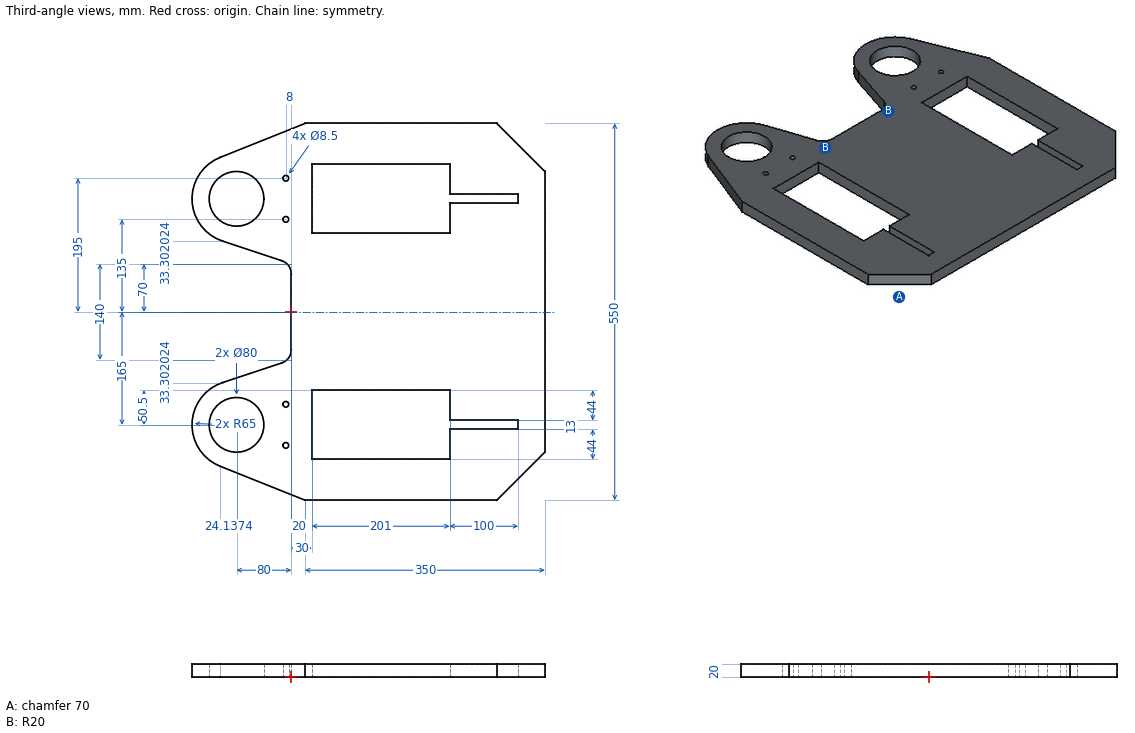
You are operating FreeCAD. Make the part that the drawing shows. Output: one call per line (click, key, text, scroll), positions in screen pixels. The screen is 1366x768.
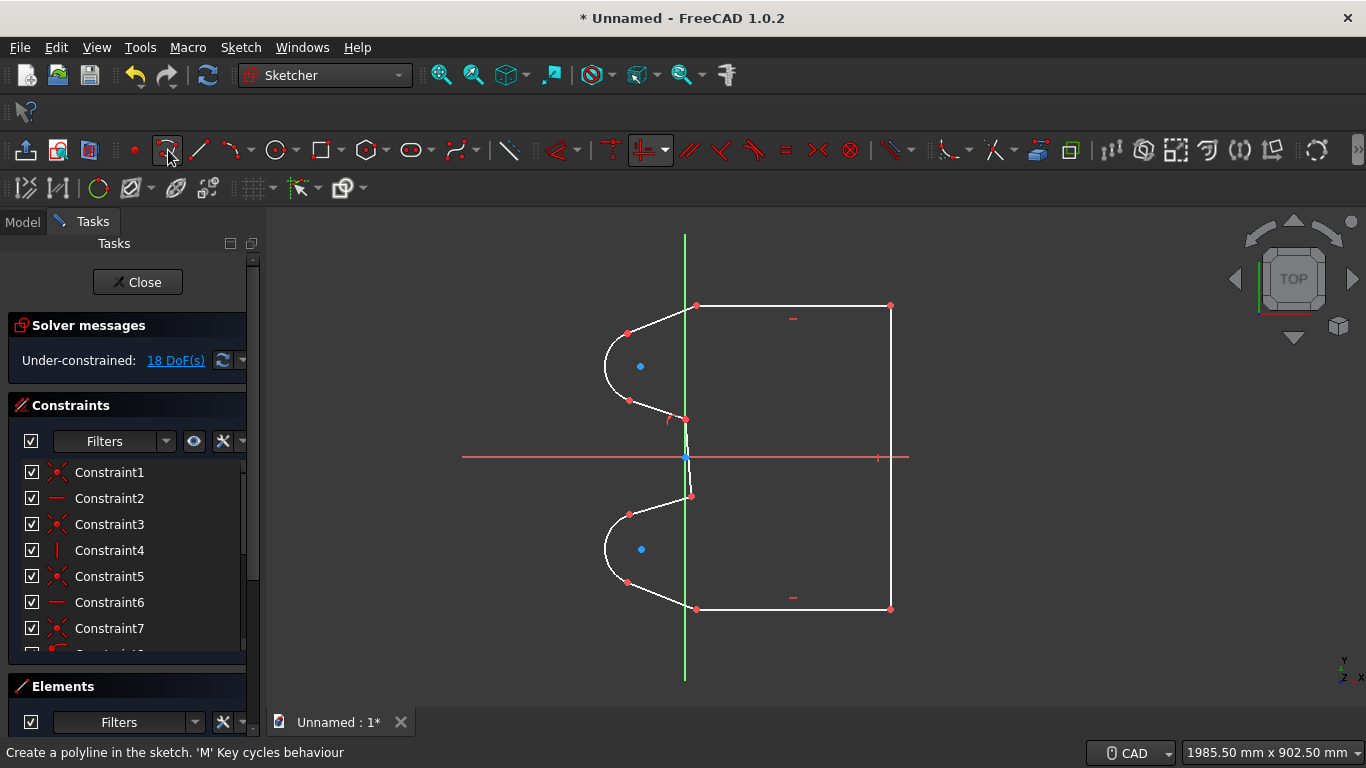
click(702, 521)
click(813, 521)
click(813, 545)
click(869, 545)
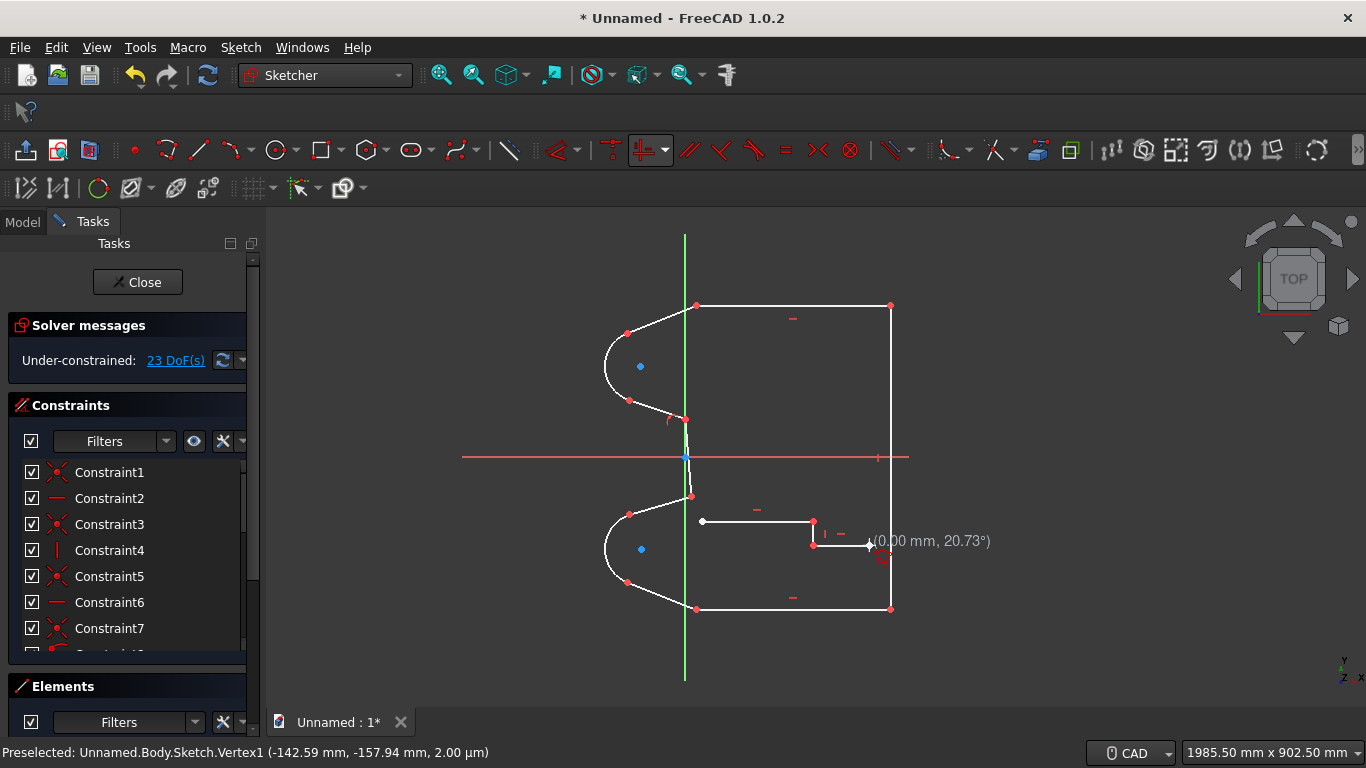
scroll(869, 552, up, 4)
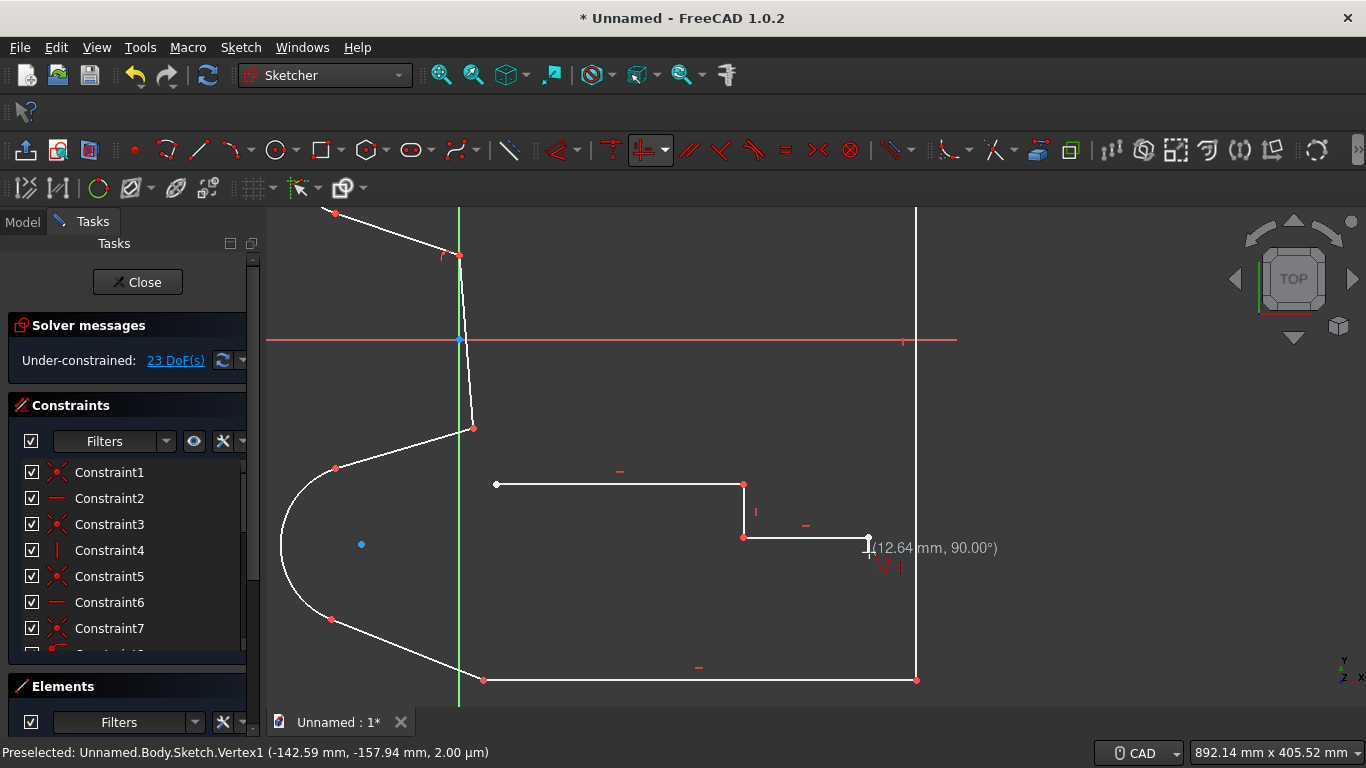
click(868, 551)
click(744, 551)
click(744, 606)
click(496, 606)
click(497, 484)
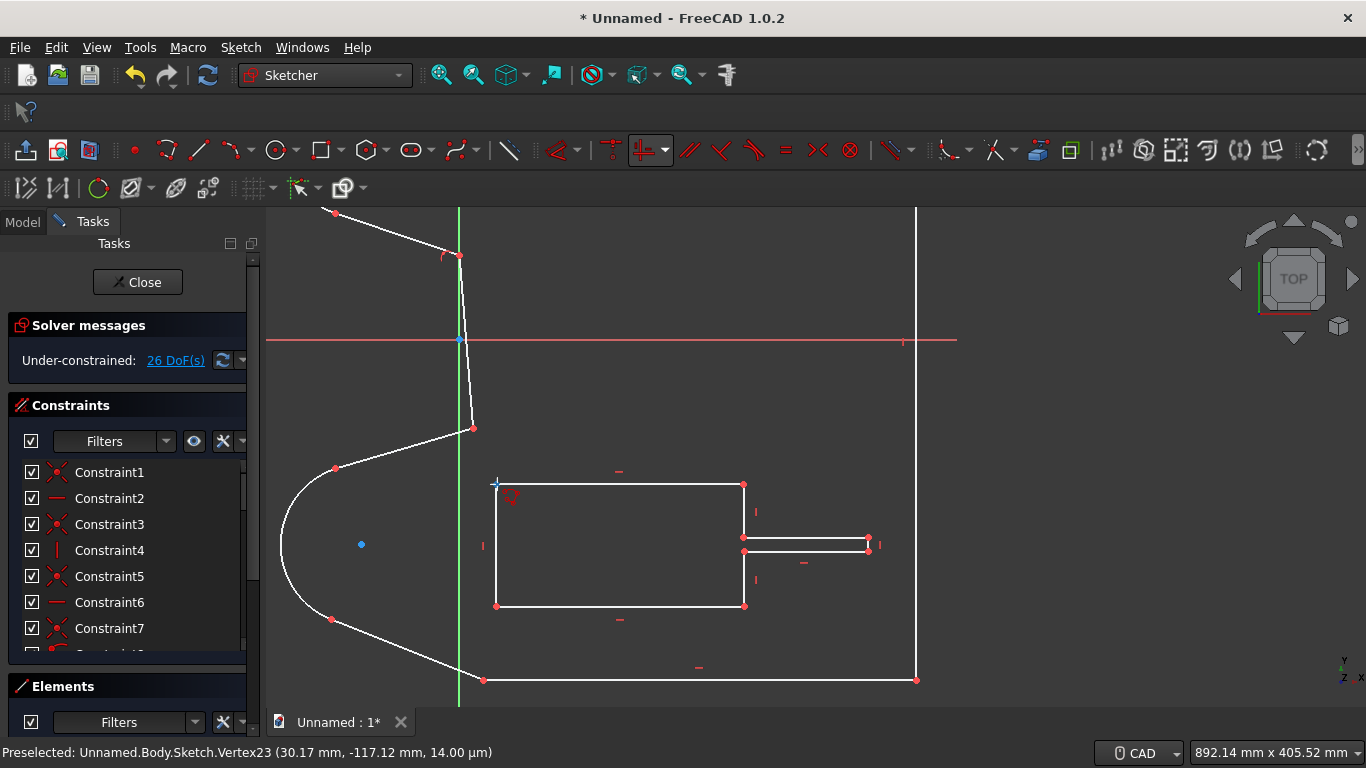
scroll(869, 552, down, 4)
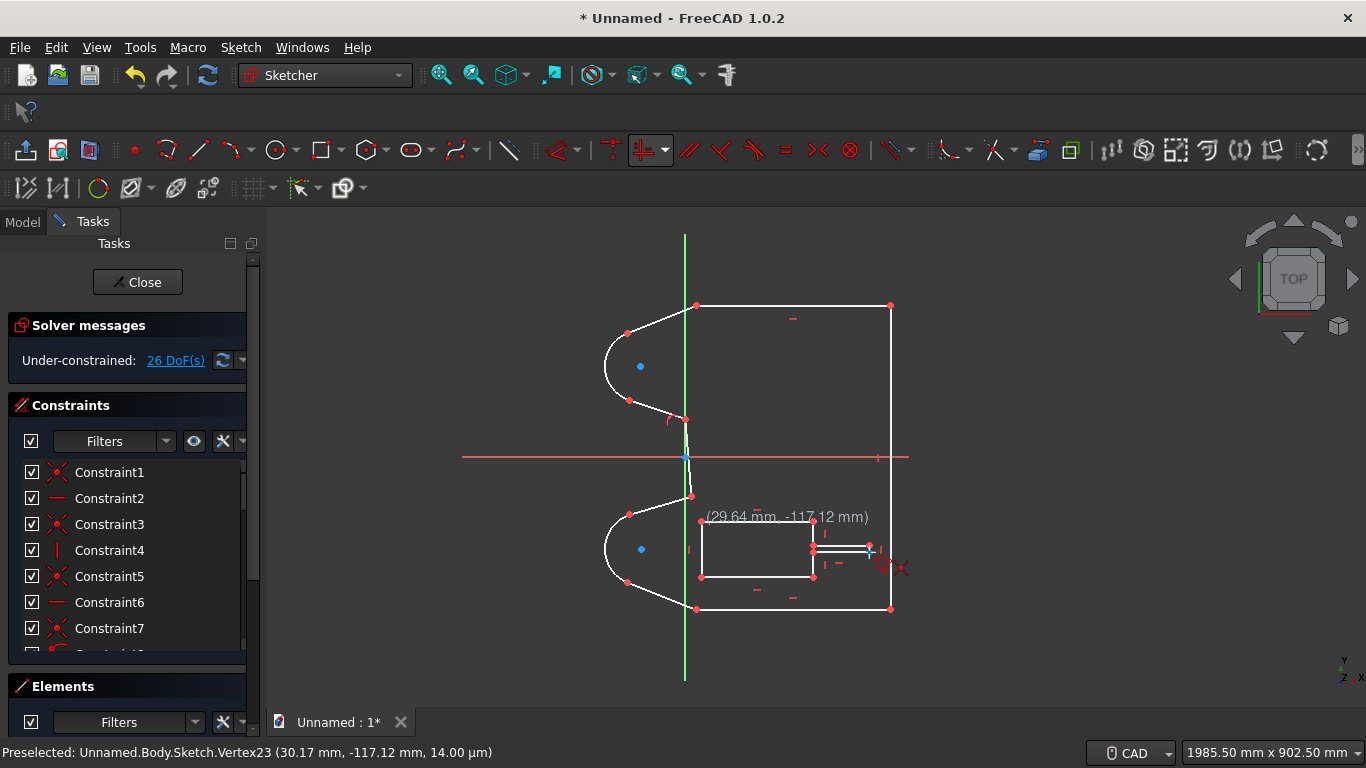
click(702, 394)
click(702, 338)
click(813, 338)
click(813, 362)
click(869, 362)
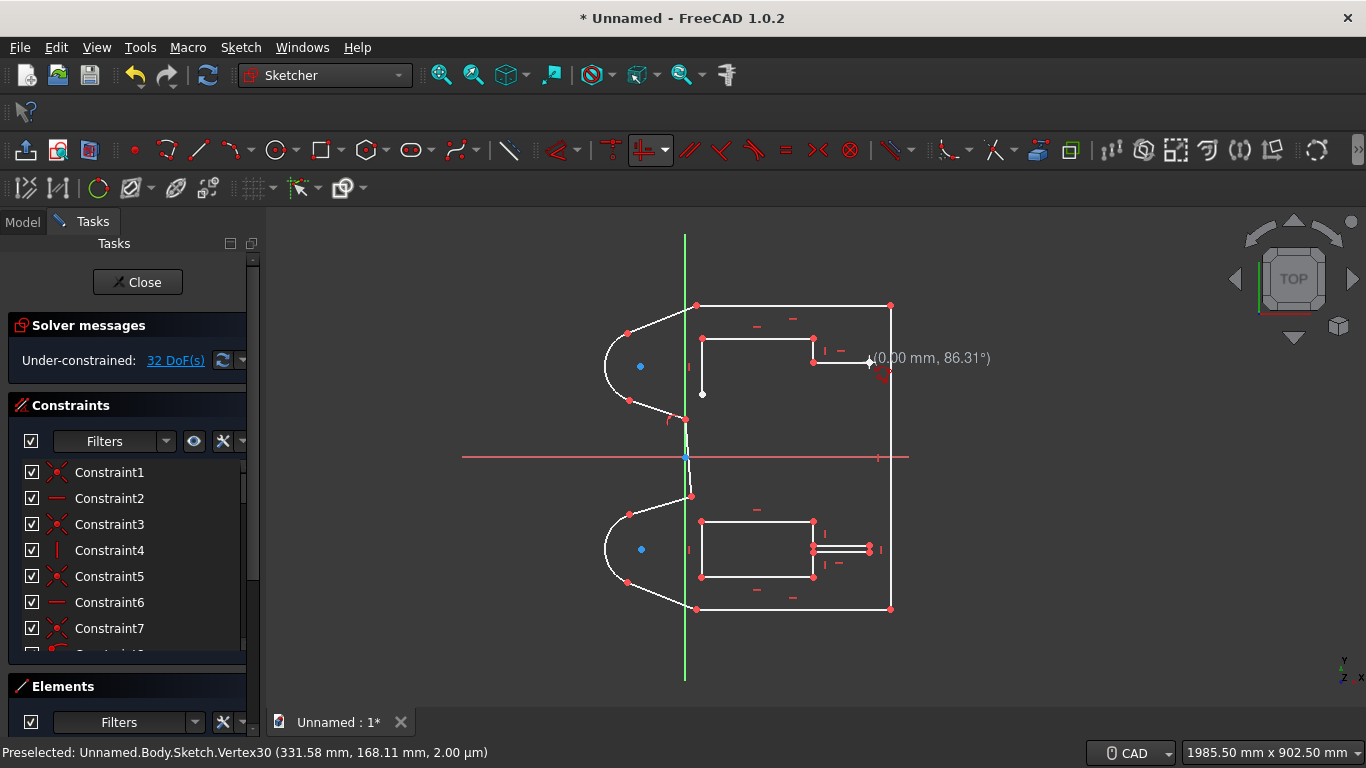
scroll(869, 369, up, 4)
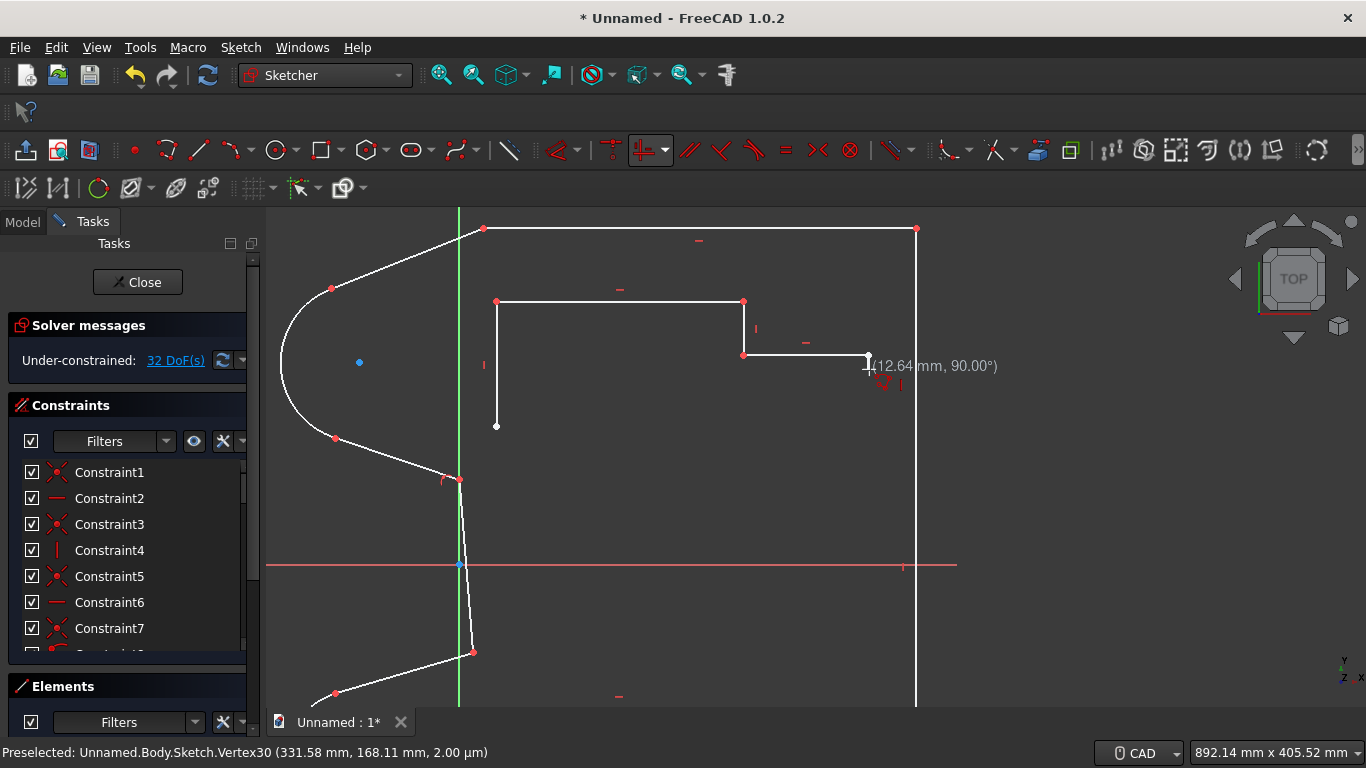
click(868, 369)
click(744, 369)
click(744, 424)
click(497, 426)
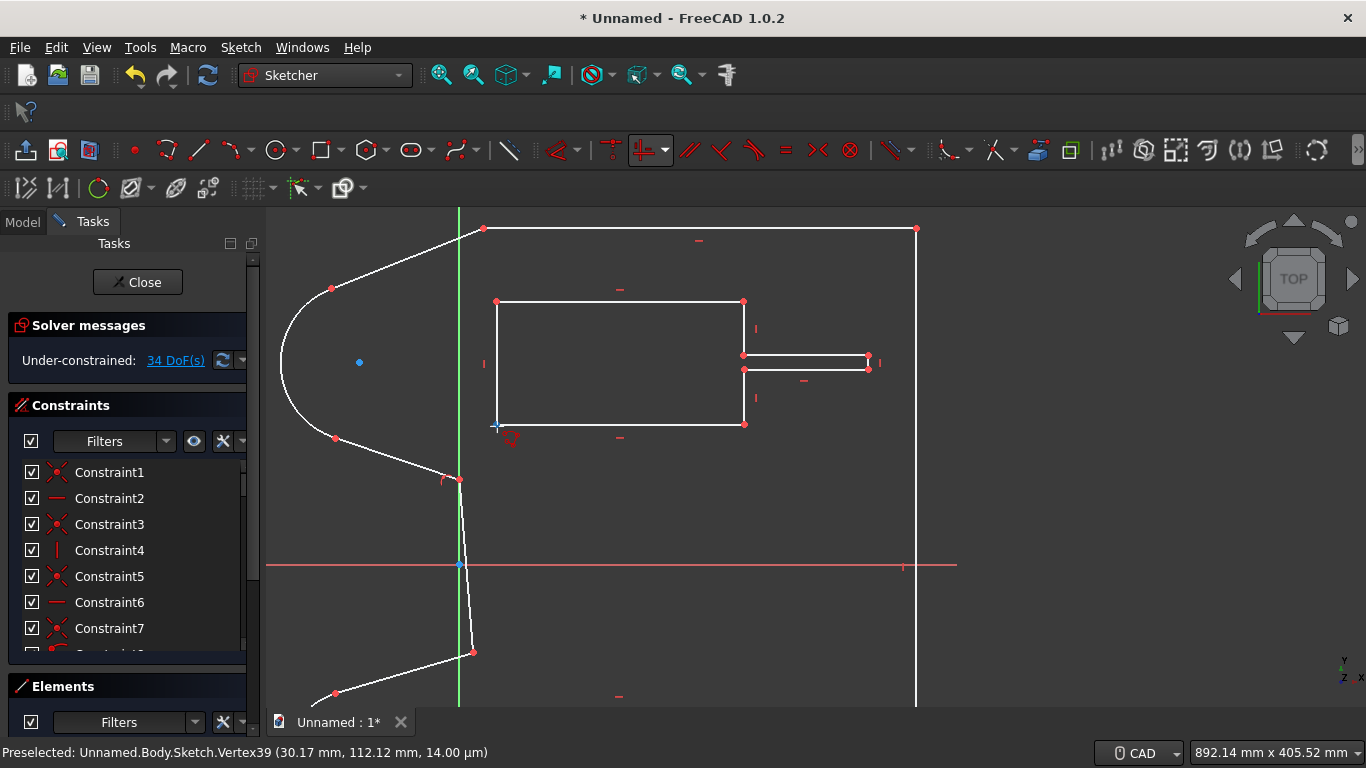
click(276, 150)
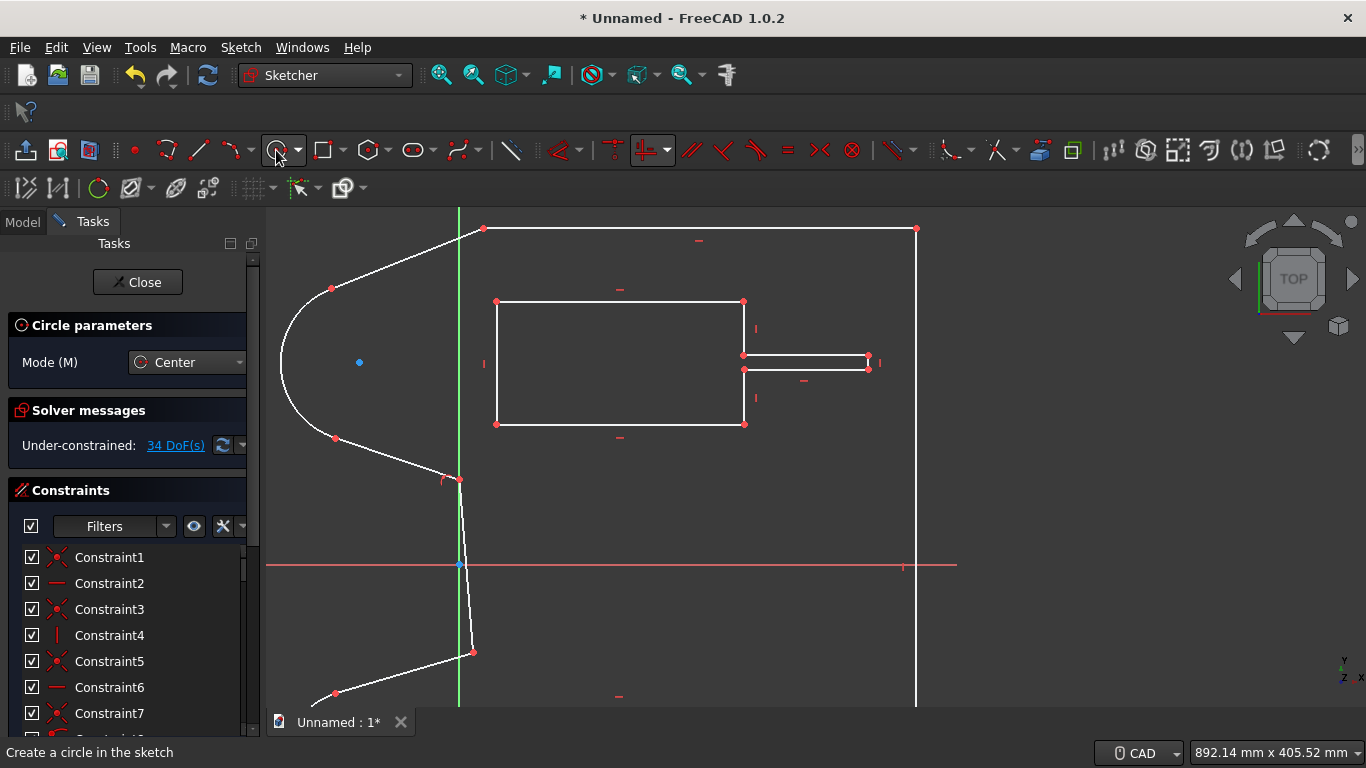
scroll(869, 369, down, 4)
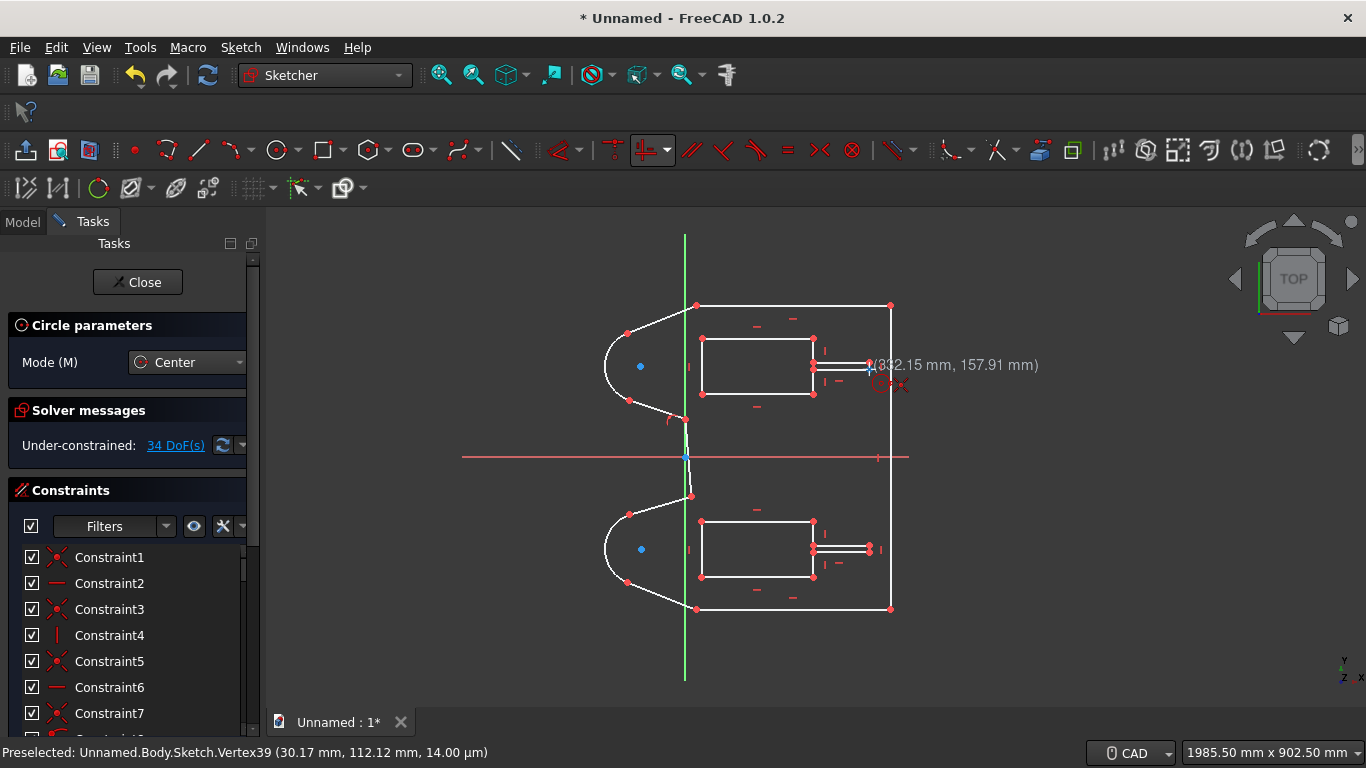
click(641, 549)
move(657, 533)